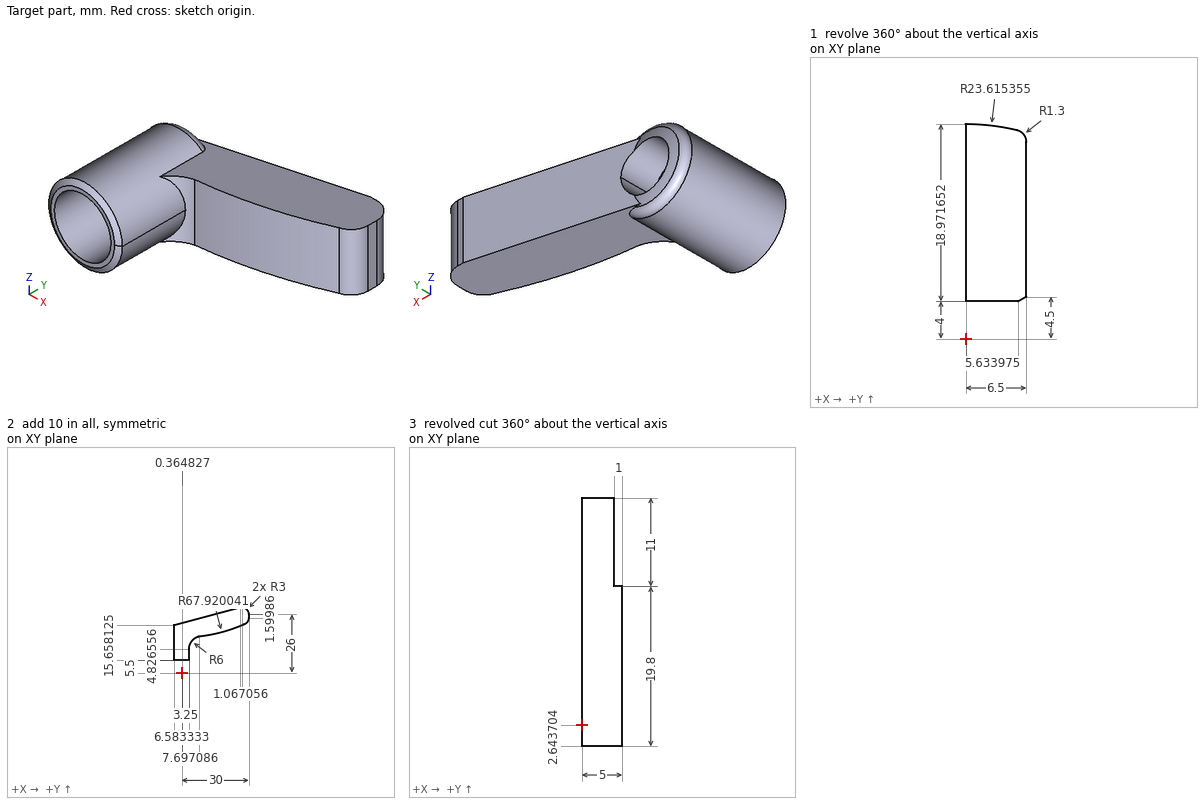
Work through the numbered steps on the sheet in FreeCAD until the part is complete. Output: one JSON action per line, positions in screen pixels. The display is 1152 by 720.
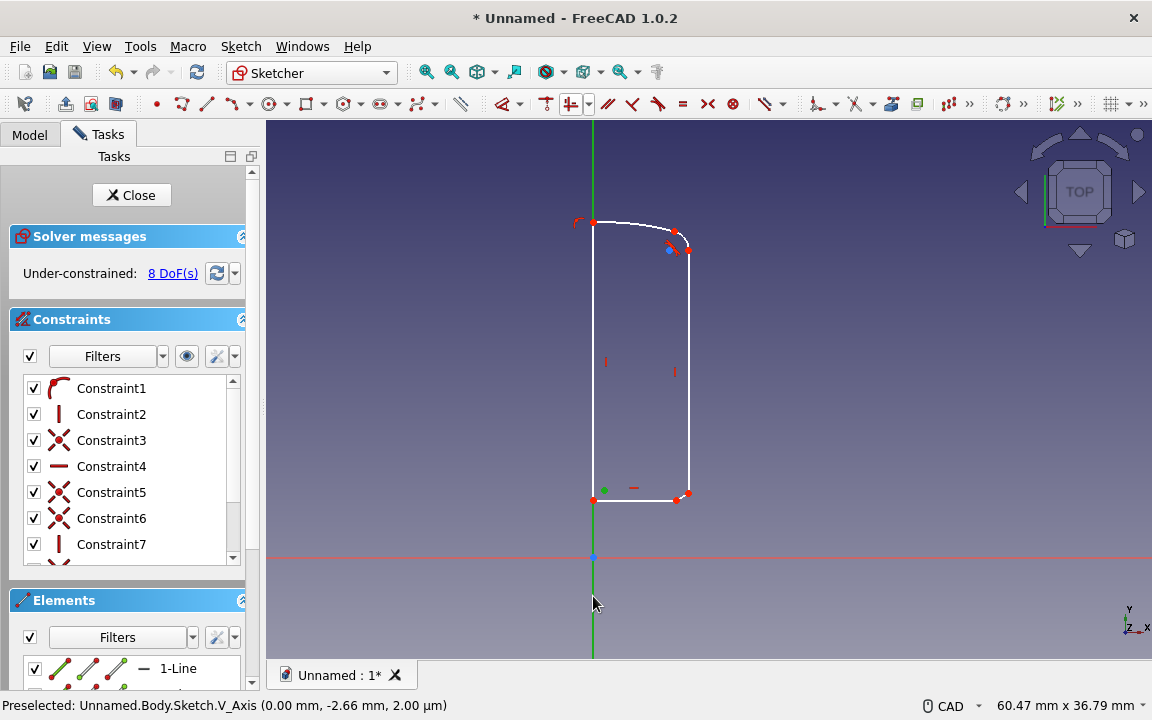
{"action": "left_click", "coordinate": [546, 104]}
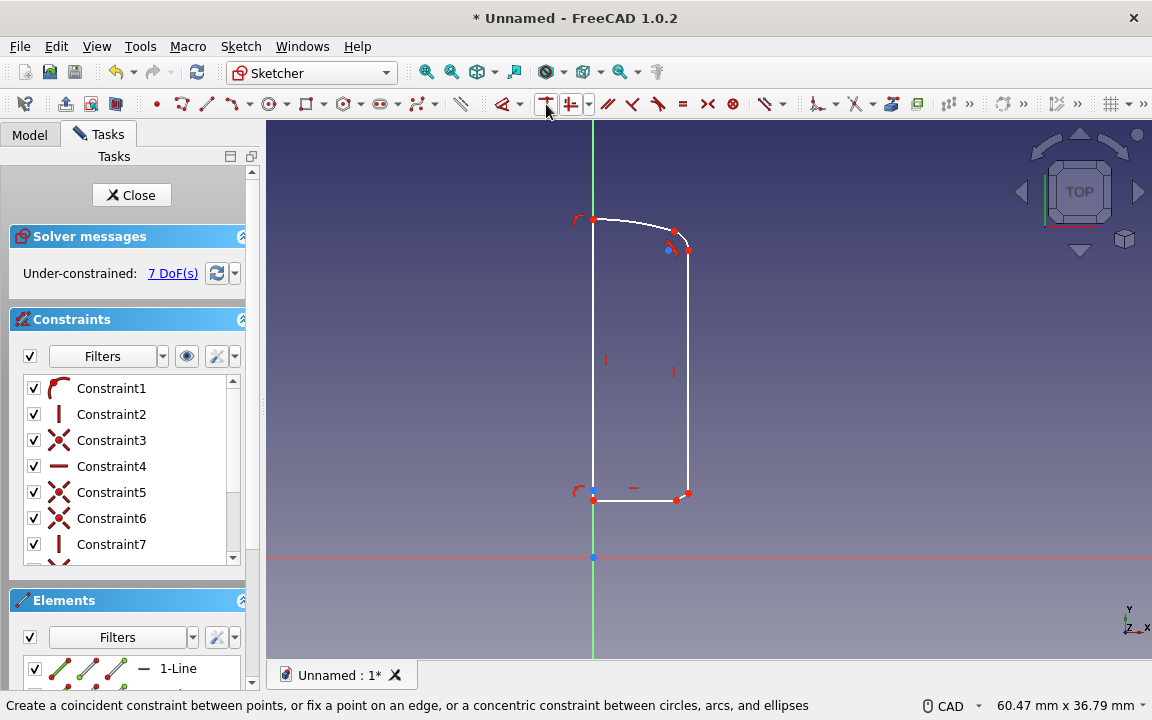
{"action": "key", "text": "d"}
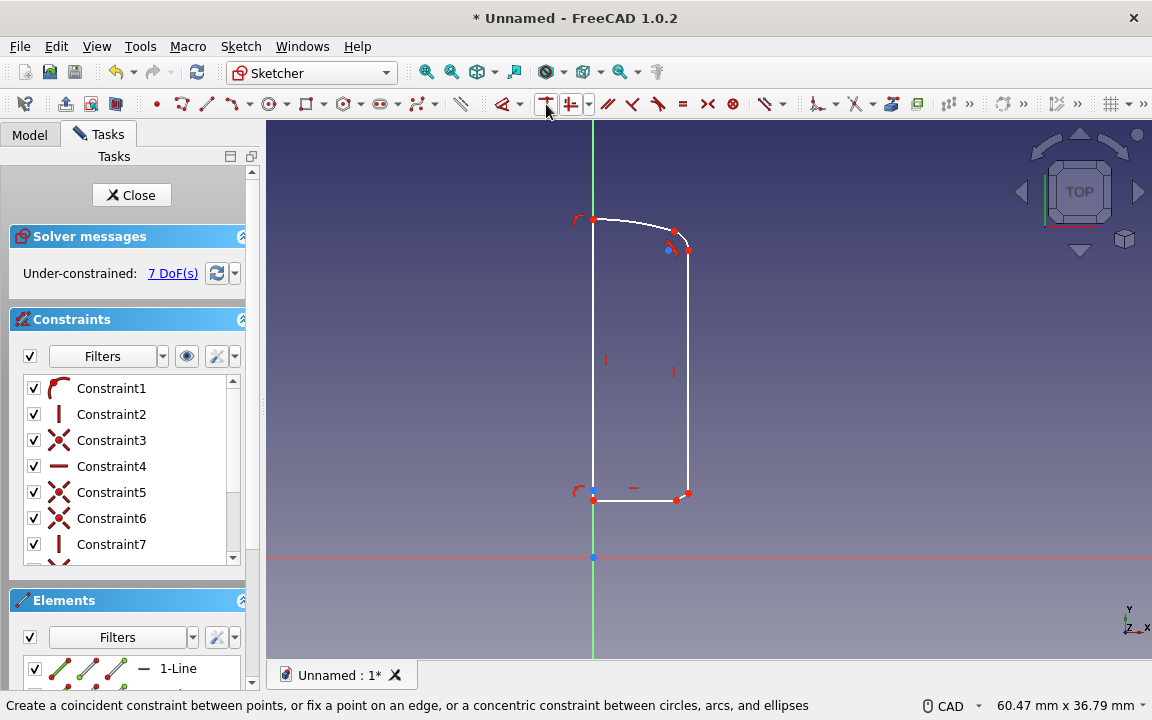
{"action": "scroll", "coordinate": [684, 239], "scroll_direction": "up", "scroll_amount": 4}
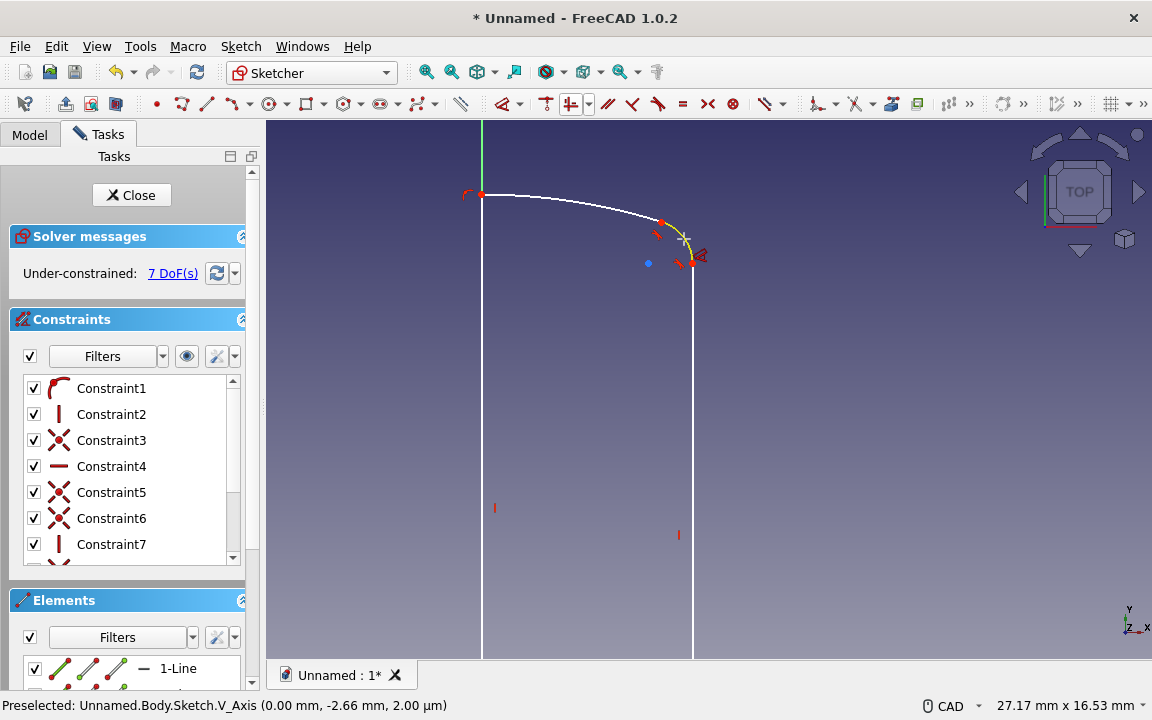
{"action": "left_click", "coordinate": [684, 238]}
{"action": "left_click", "coordinate": [710, 219]}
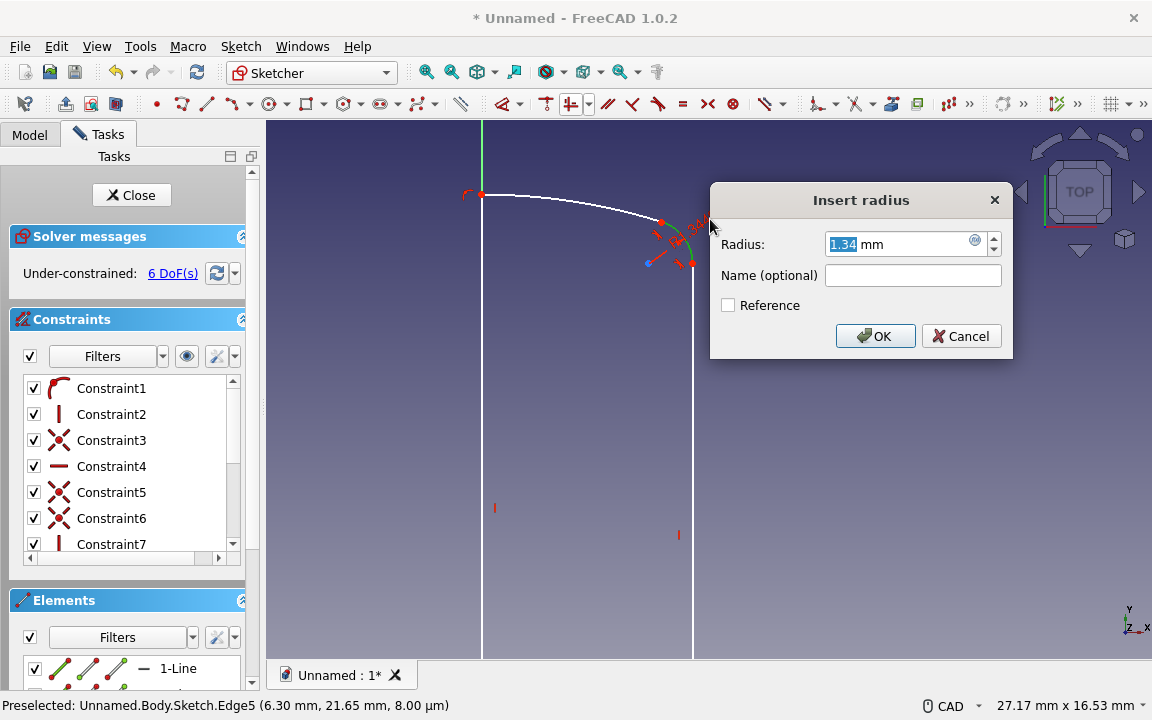
{"action": "type", "text": "1.3"}
{"action": "key", "text": "Return"}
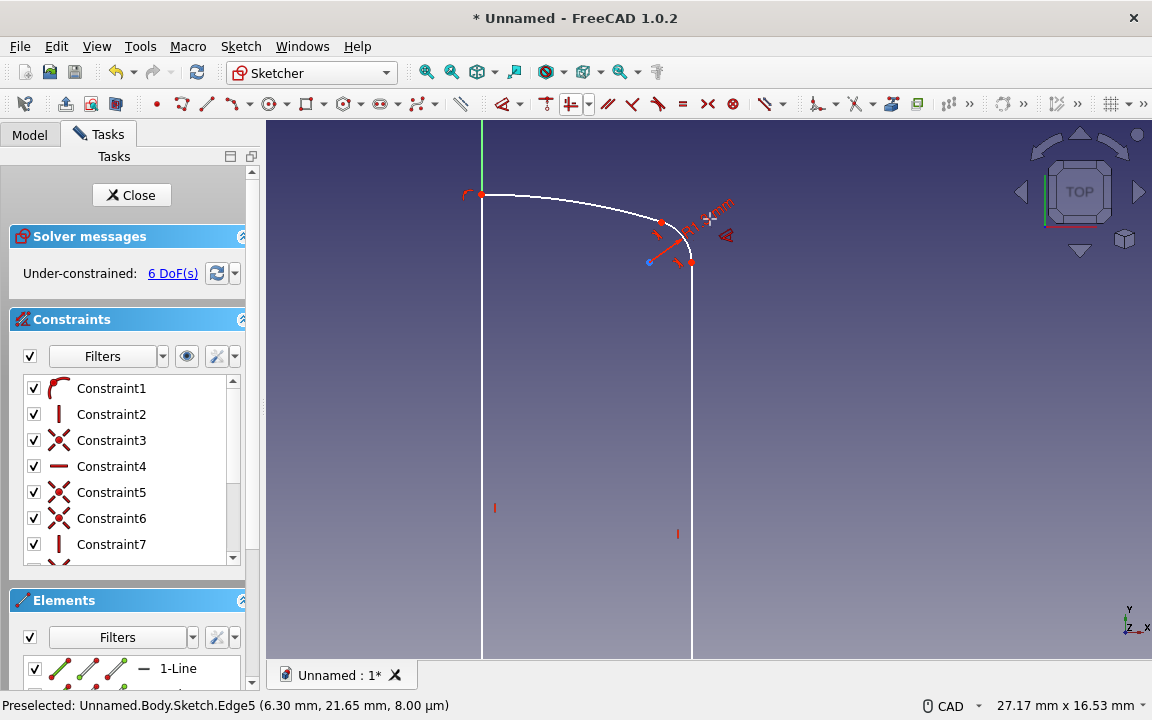
{"action": "left_click", "coordinate": [609, 208]}
{"action": "left_click", "coordinate": [616, 177]}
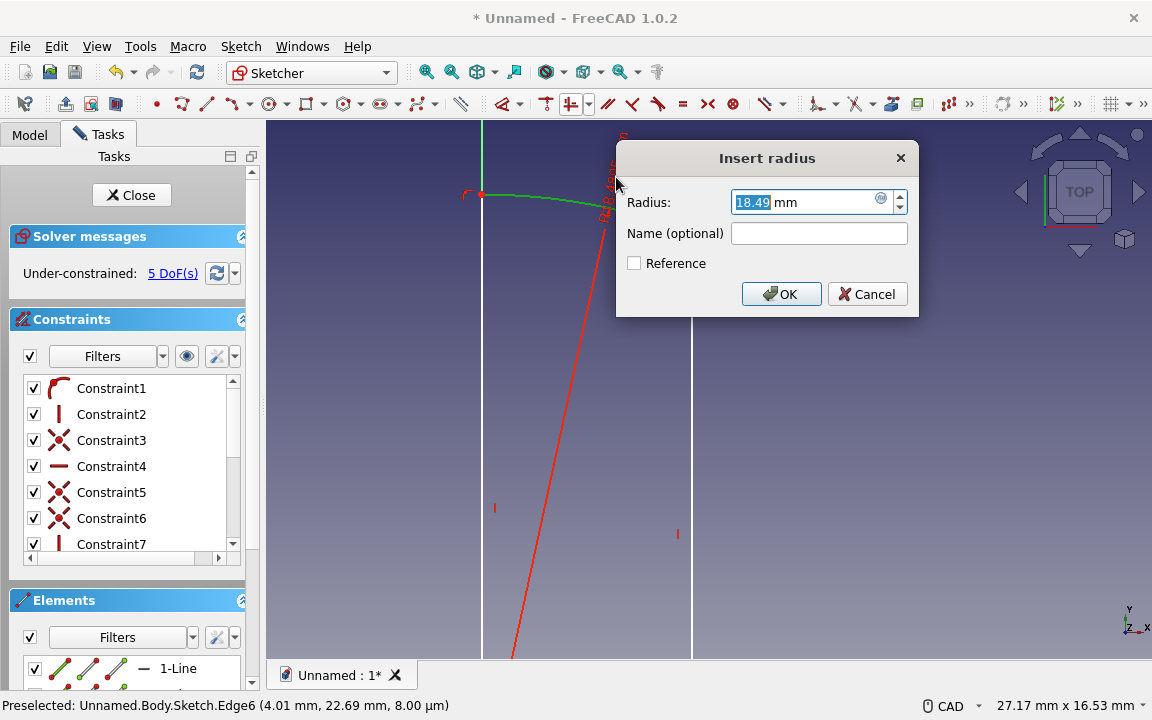
{"action": "type", "text": "23.615355"}
{"action": "key", "text": "Return"}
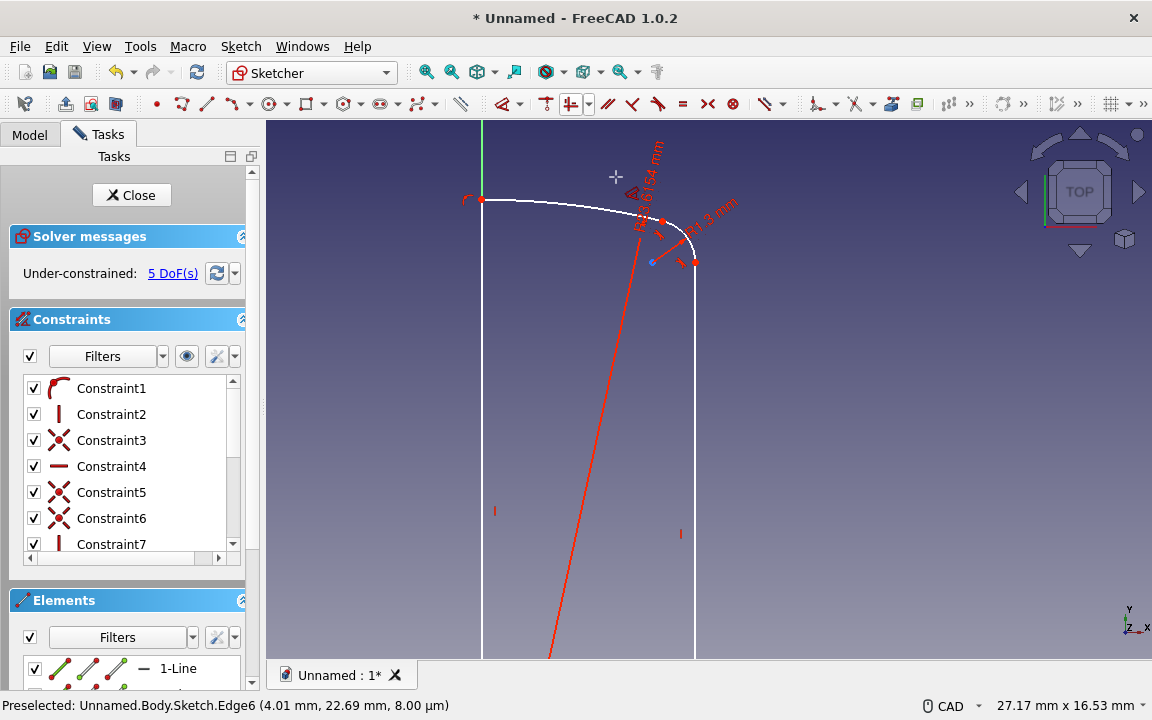
{"action": "scroll", "coordinate": [683, 239], "scroll_direction": "down", "scroll_amount": 4}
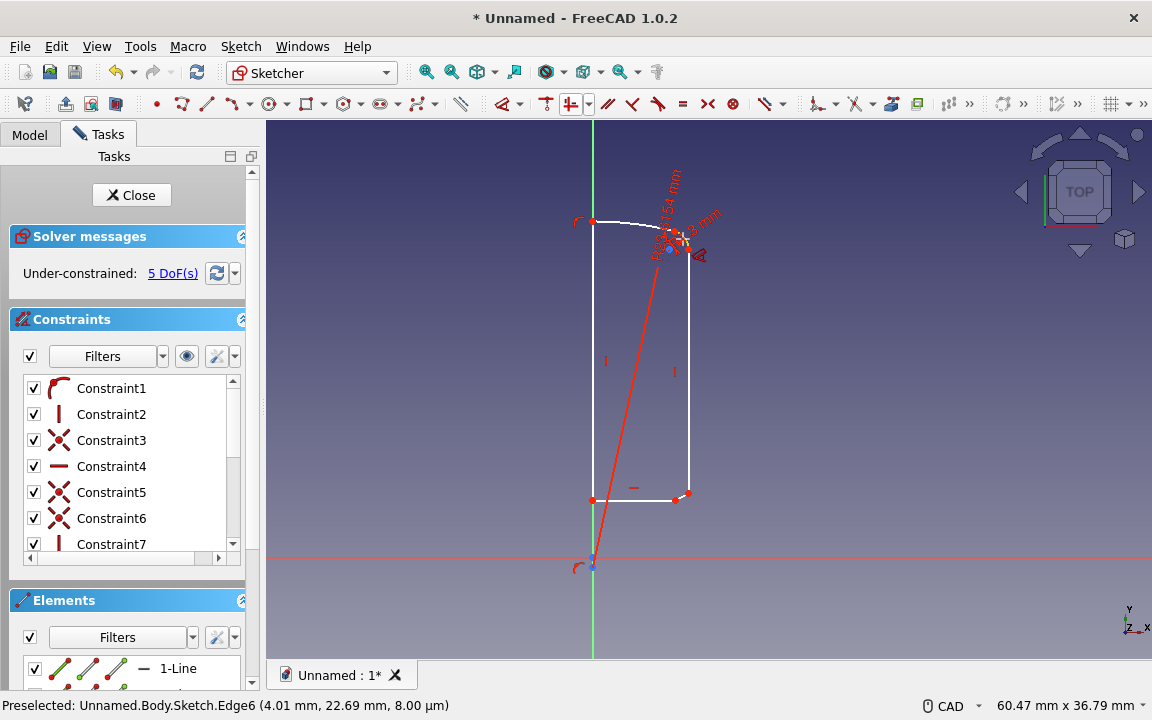
{"action": "left_click", "coordinate": [593, 501]}
{"action": "left_click", "coordinate": [559, 529]}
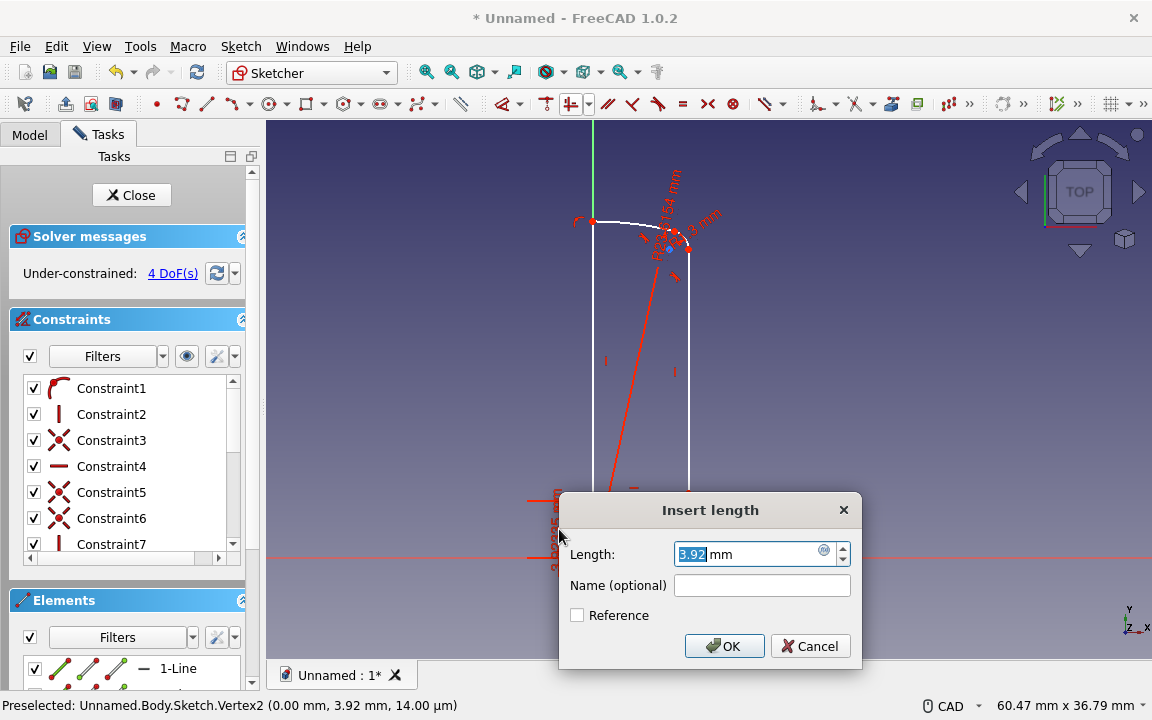
{"action": "type", "text": "4"}
{"action": "key", "text": "Return"}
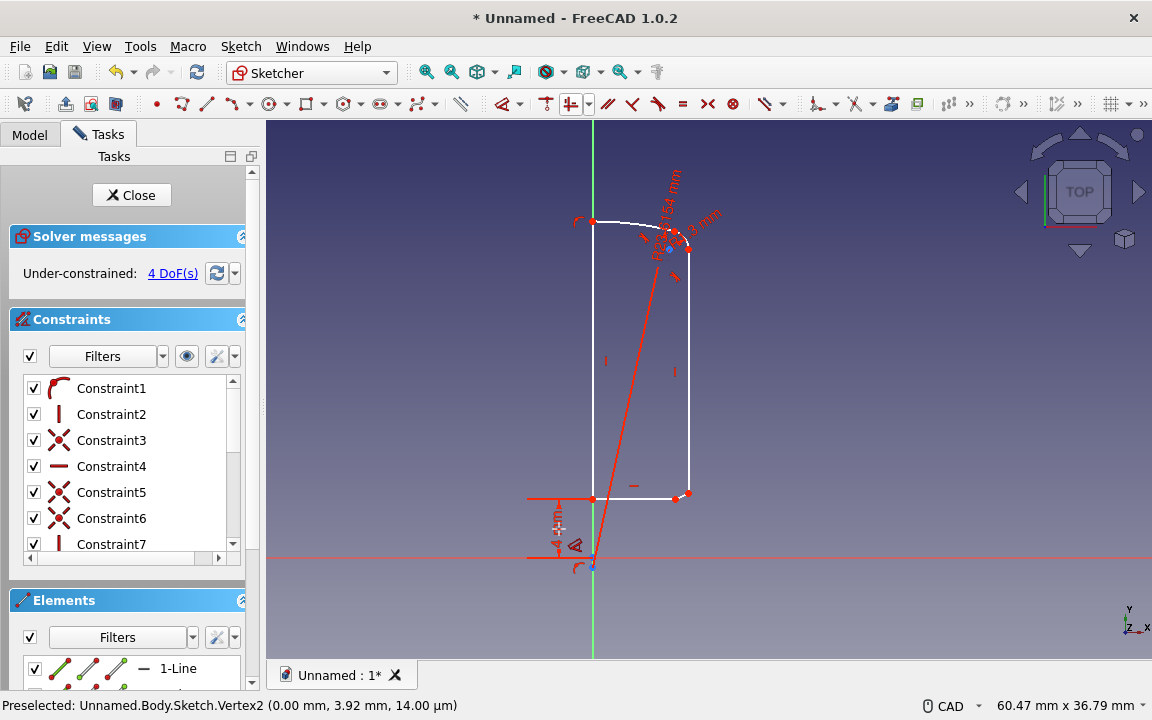
{"action": "left_click", "coordinate": [689, 494]}
{"action": "left_click", "coordinate": [641, 592]}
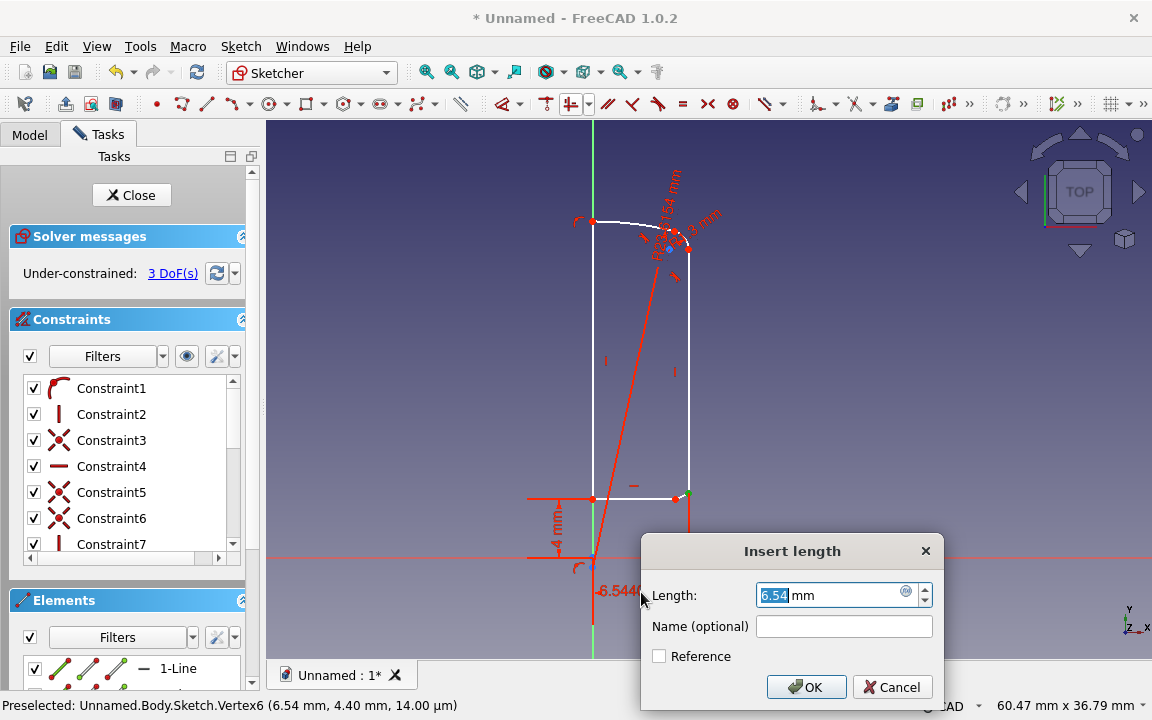
{"action": "type", "text": "6.5"}
{"action": "key", "text": "Return"}